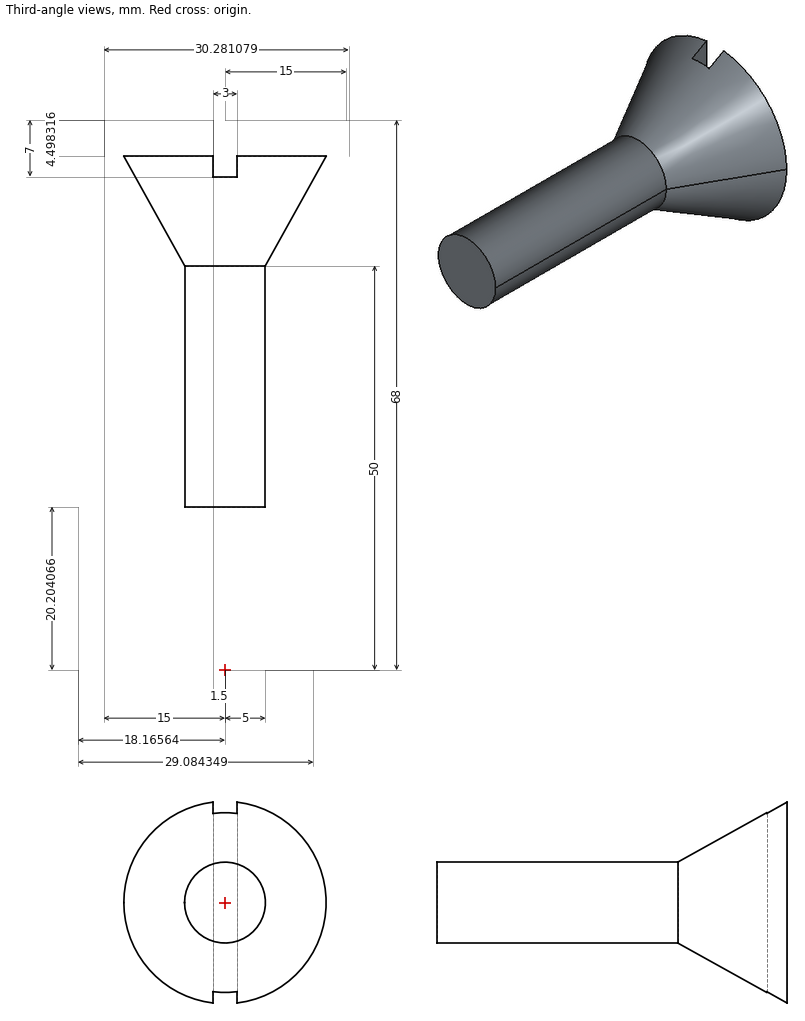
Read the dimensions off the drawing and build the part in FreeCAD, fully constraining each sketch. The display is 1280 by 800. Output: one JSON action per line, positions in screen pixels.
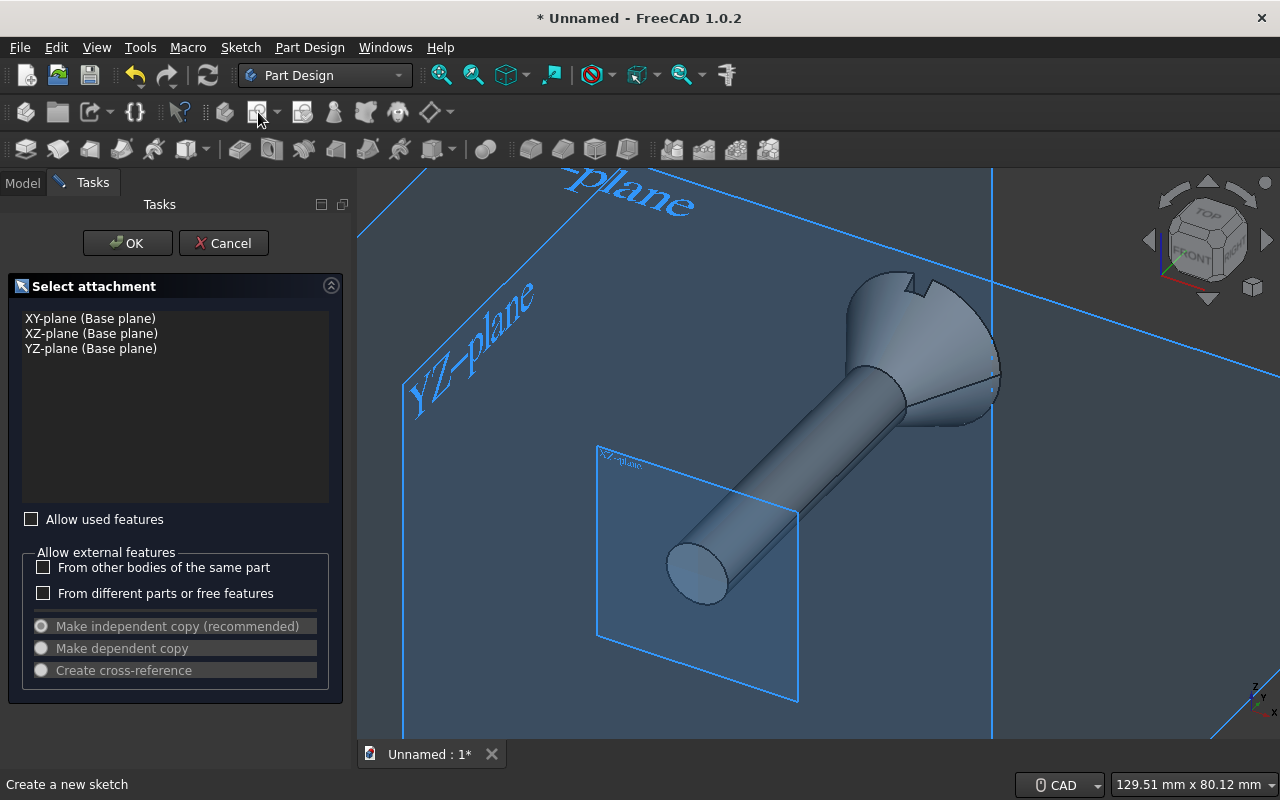
{"action": "left_click", "coordinate": [82, 318]}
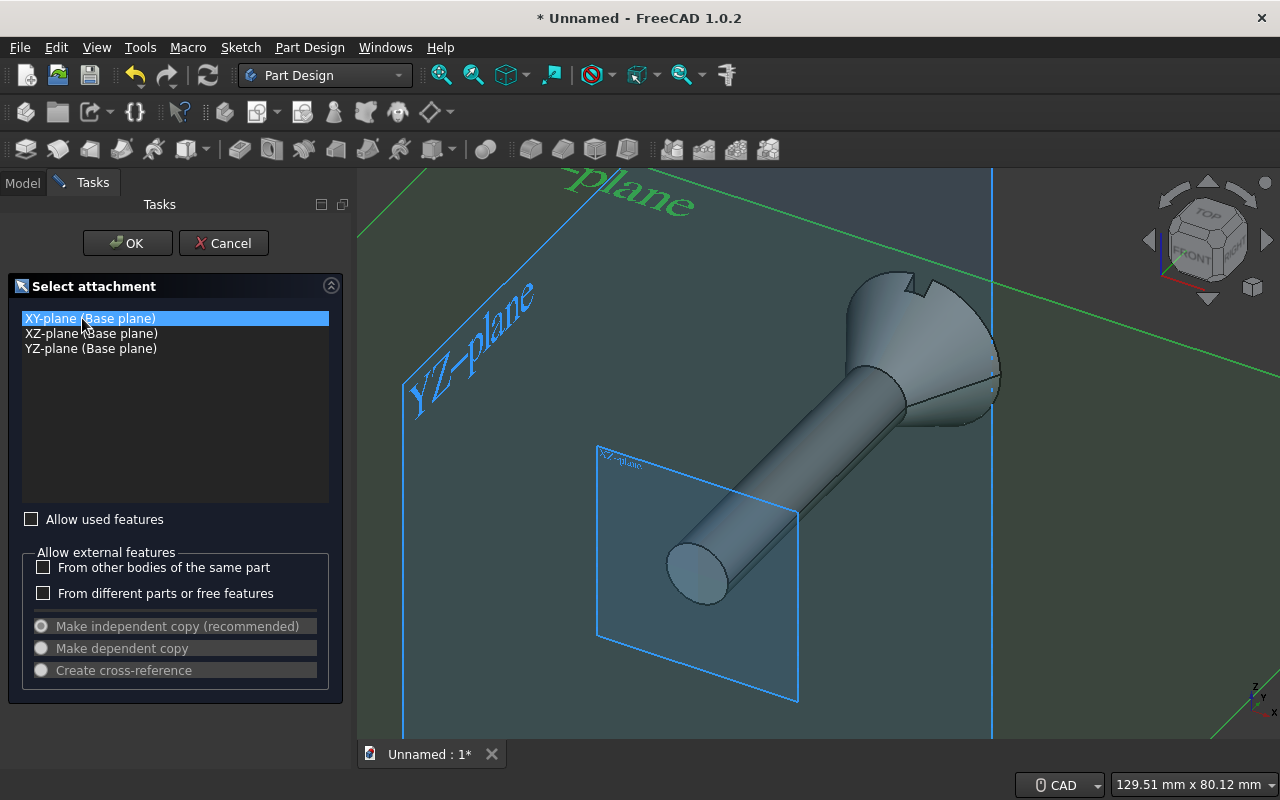
{"action": "left_click", "coordinate": [128, 243]}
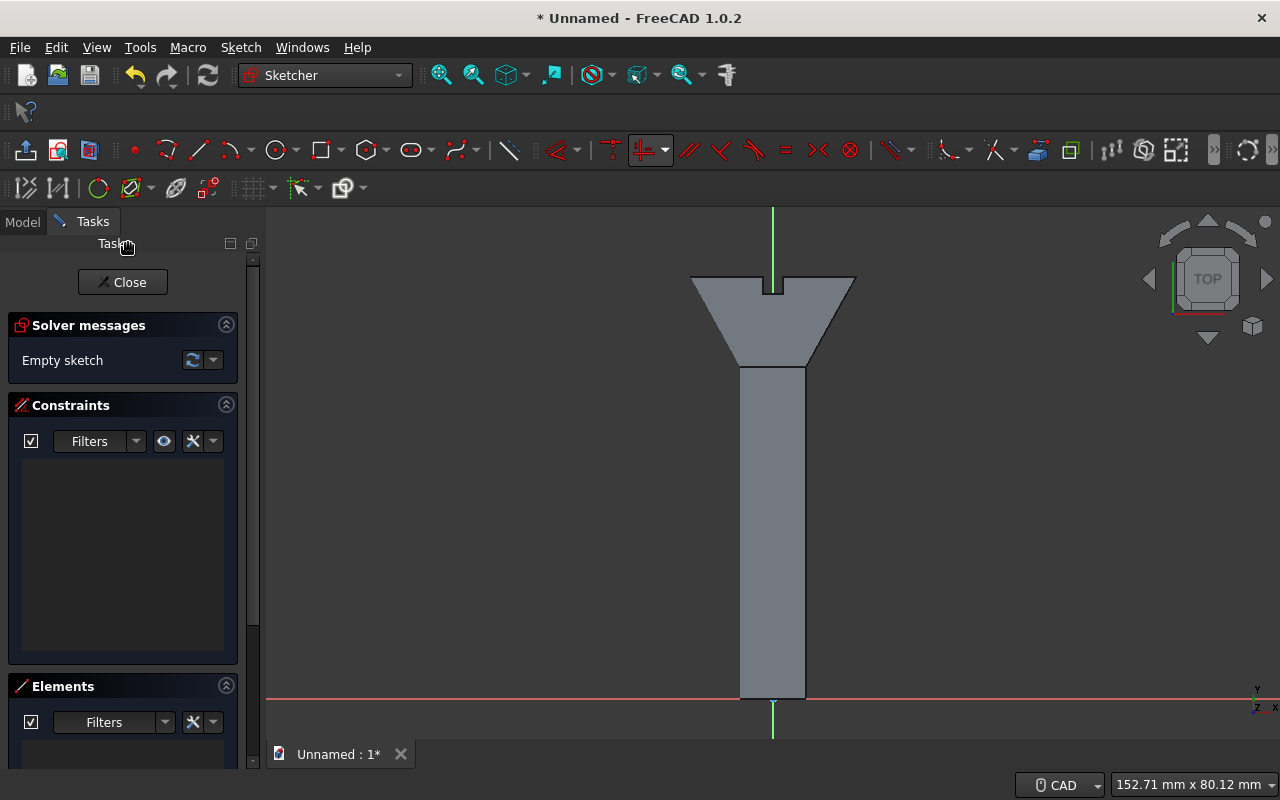
{"action": "left_click", "coordinate": [90, 150]}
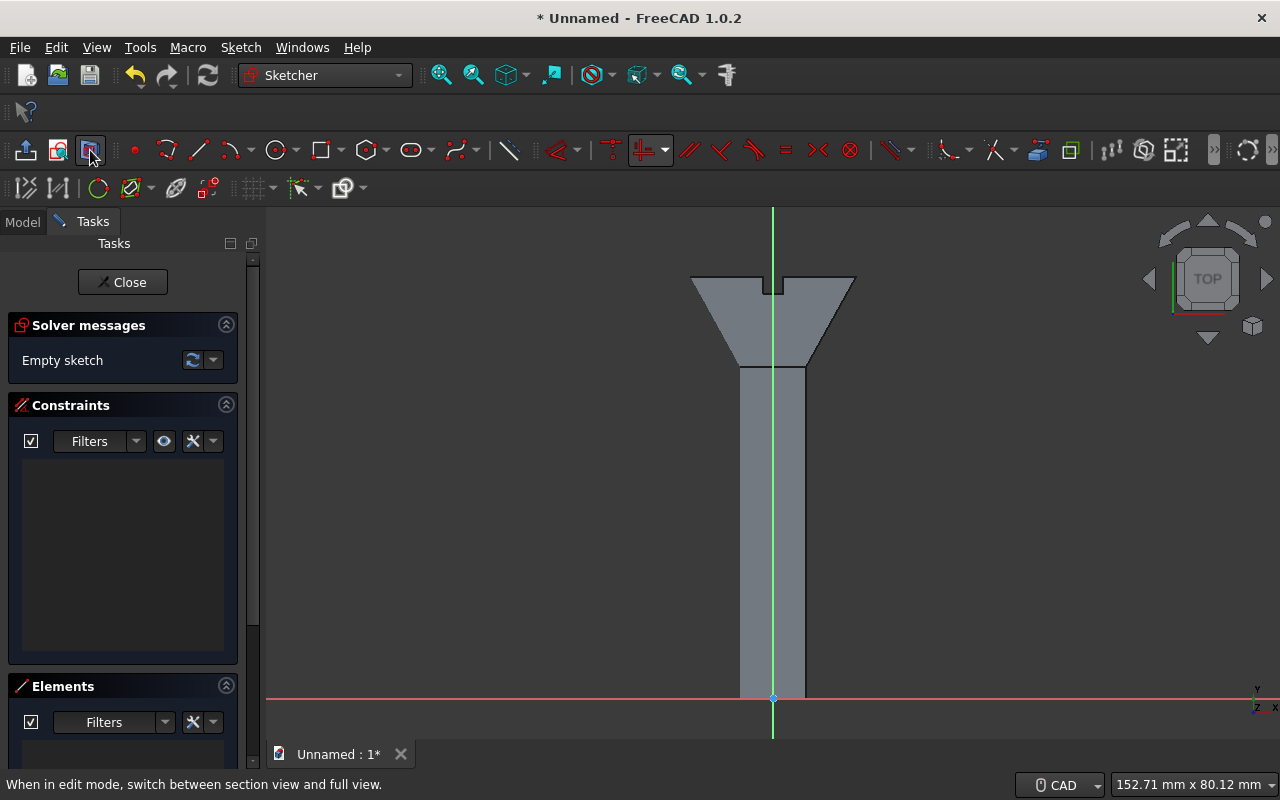
{"action": "scroll", "coordinate": [775, 711], "scroll_direction": "up", "scroll_amount": 5}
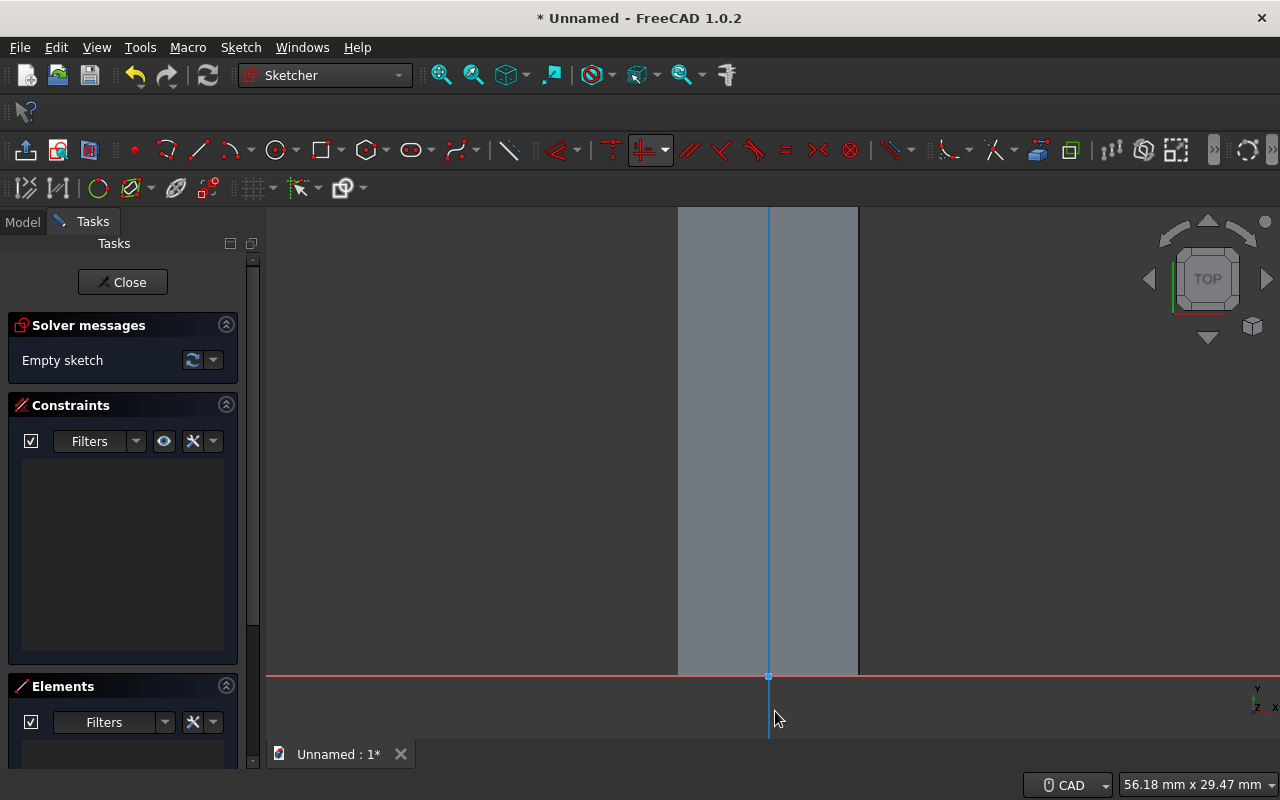
{"action": "key", "text": "g r"}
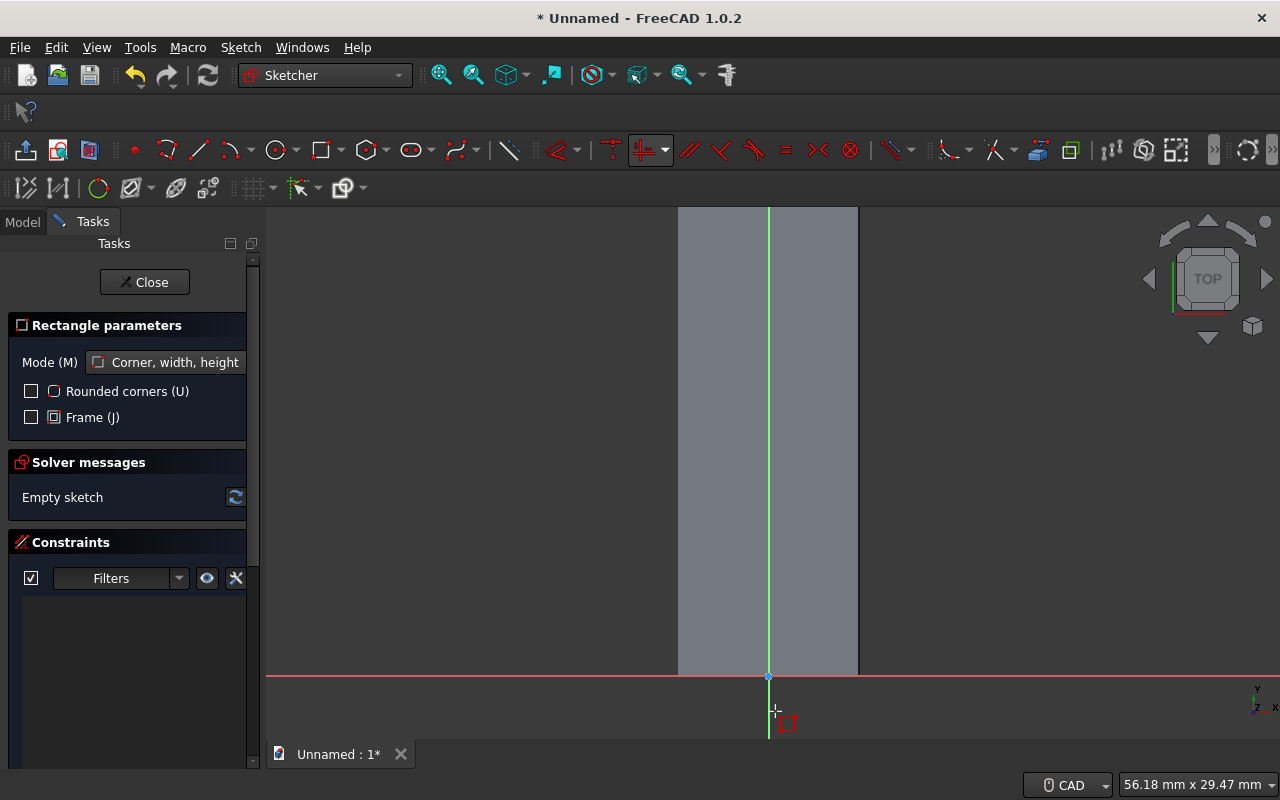
{"action": "left_click", "coordinate": [441, 311]}
{"action": "left_click", "coordinate": [966, 676]}
{"action": "key", "text": "Escape"}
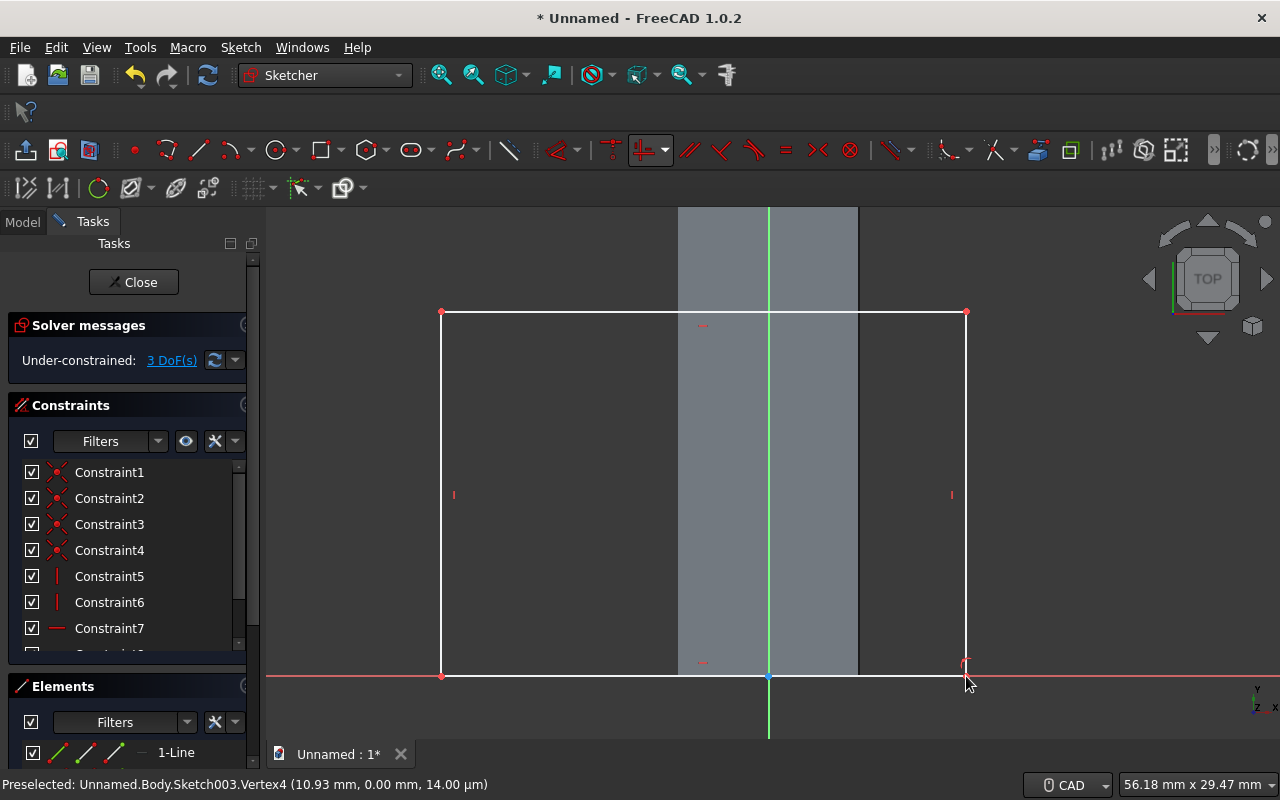
{"action": "key", "text": "d"}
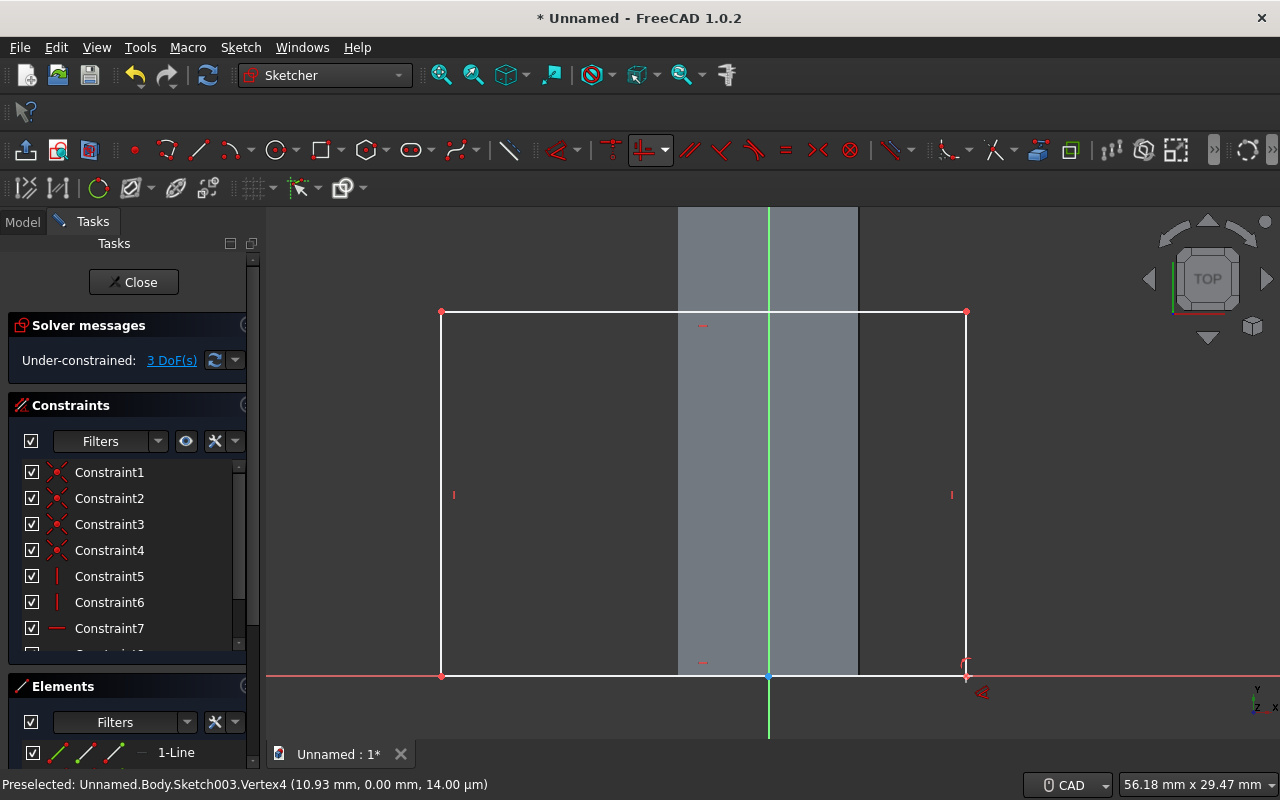
{"action": "left_click", "coordinate": [441, 421]}
{"action": "left_click", "coordinate": [407, 494]}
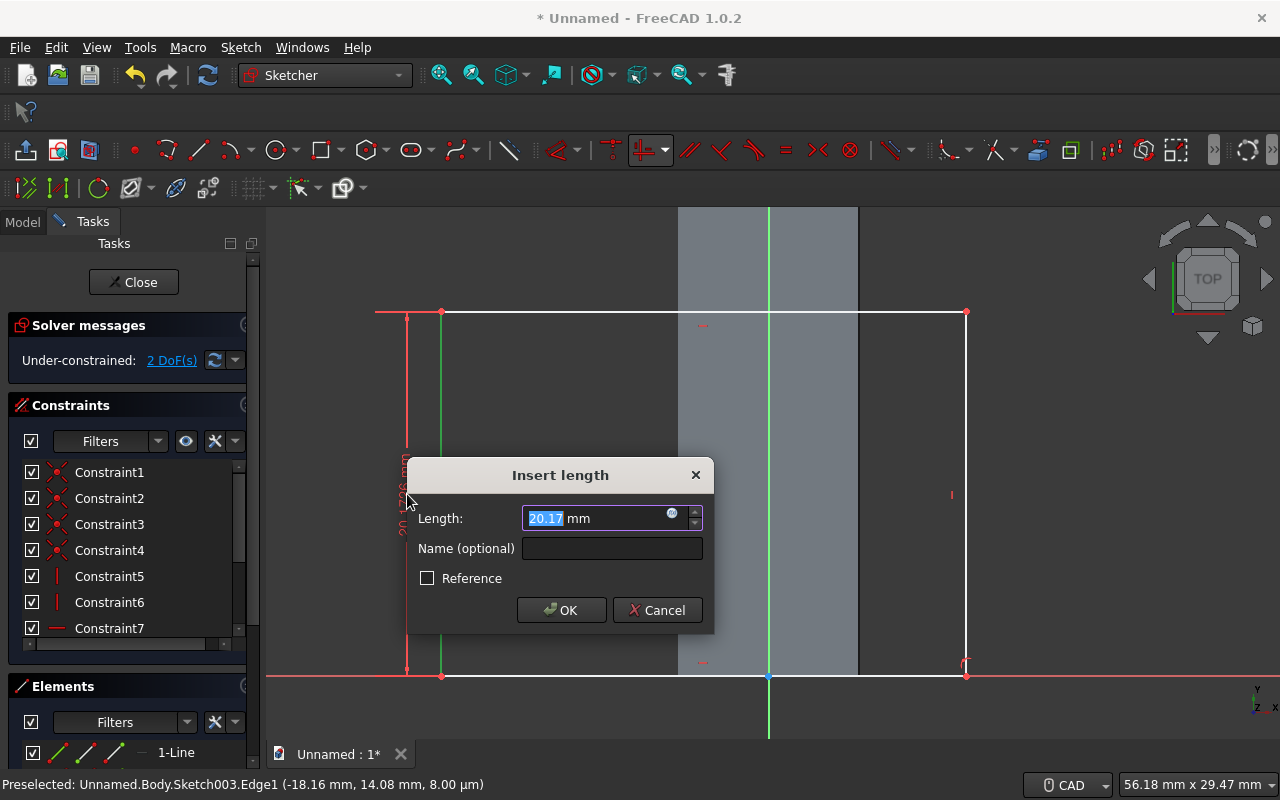
{"action": "type", "text": "20.204066"}
{"action": "key", "text": "Return"}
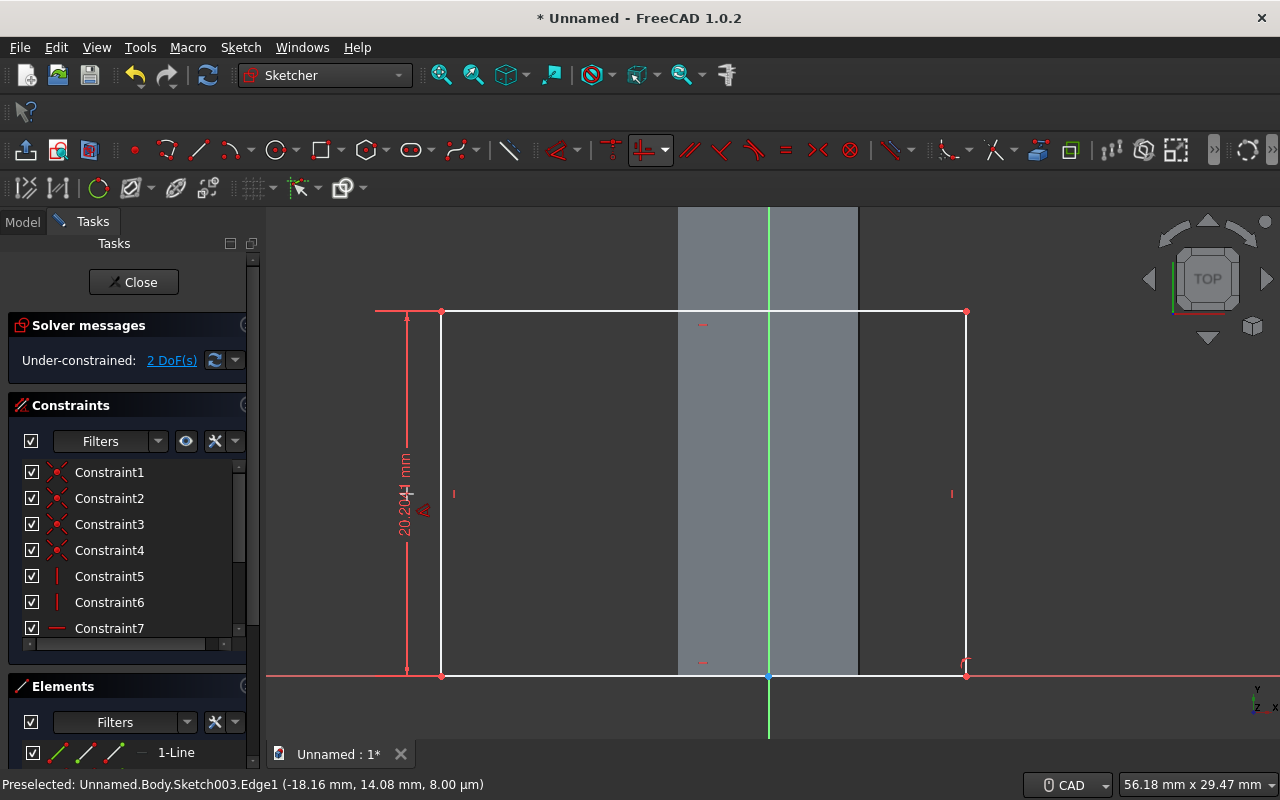
{"action": "left_click", "coordinate": [599, 676]}
{"action": "left_click", "coordinate": [704, 710]}